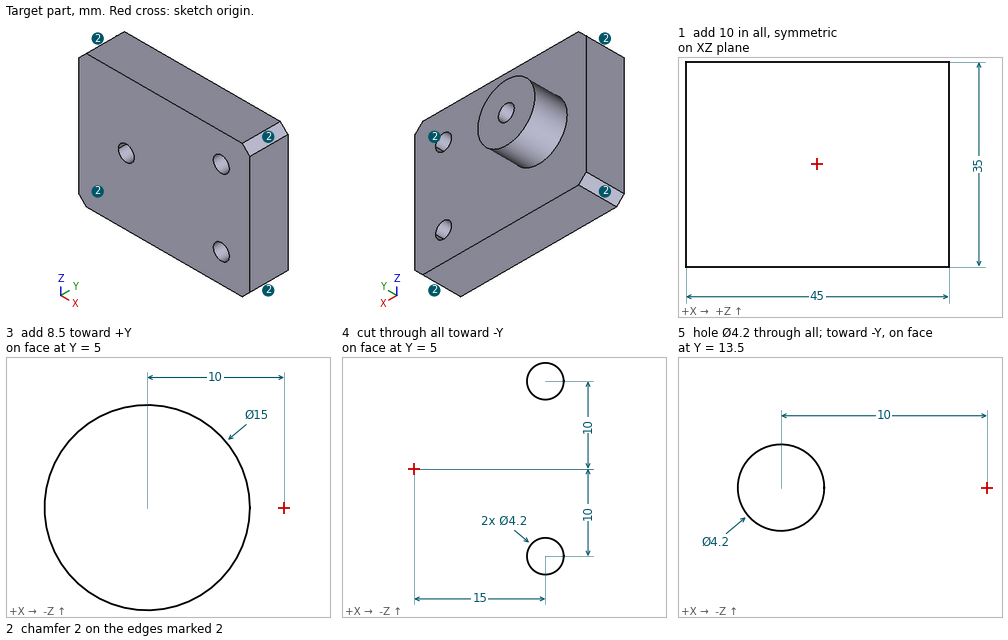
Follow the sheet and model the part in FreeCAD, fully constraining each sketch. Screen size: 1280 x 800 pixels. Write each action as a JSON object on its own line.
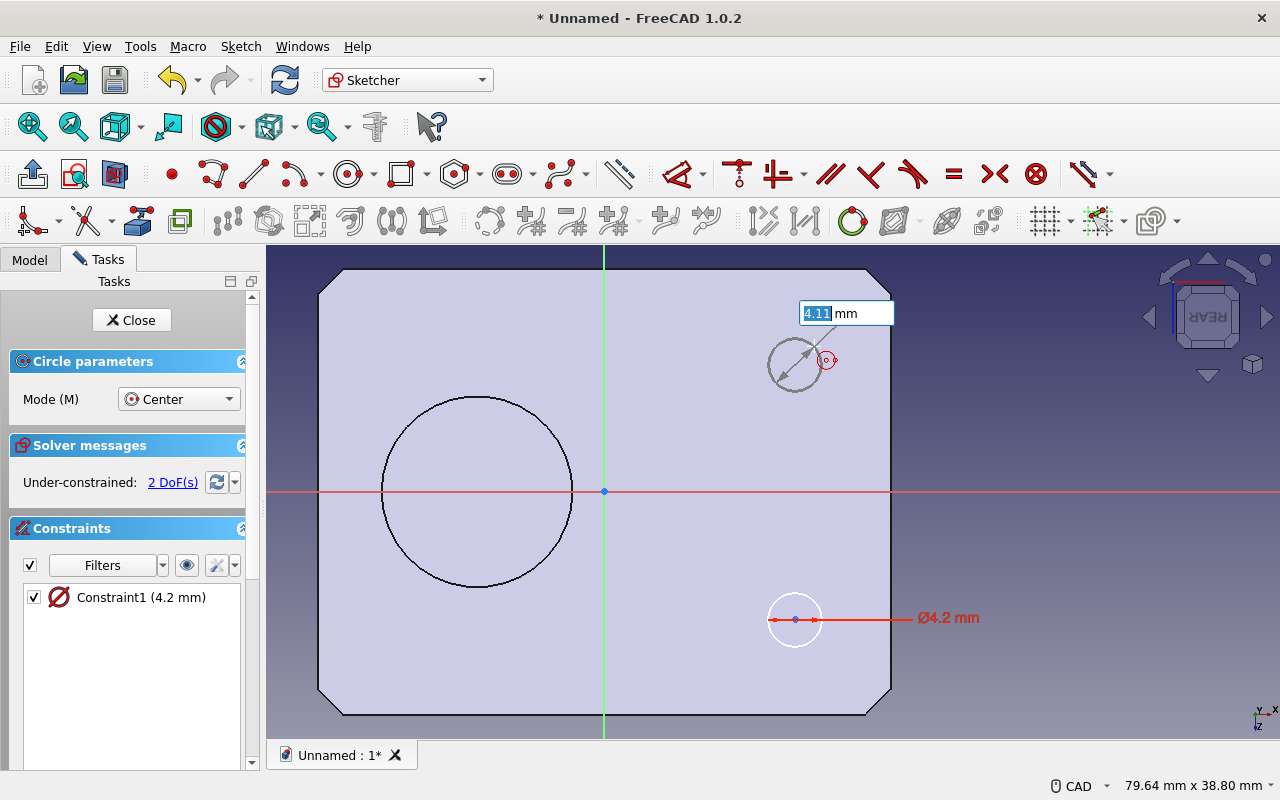
{"action": "type", "text": "4.2"}
{"action": "key", "text": "Return"}
{"action": "key", "text": "Escape"}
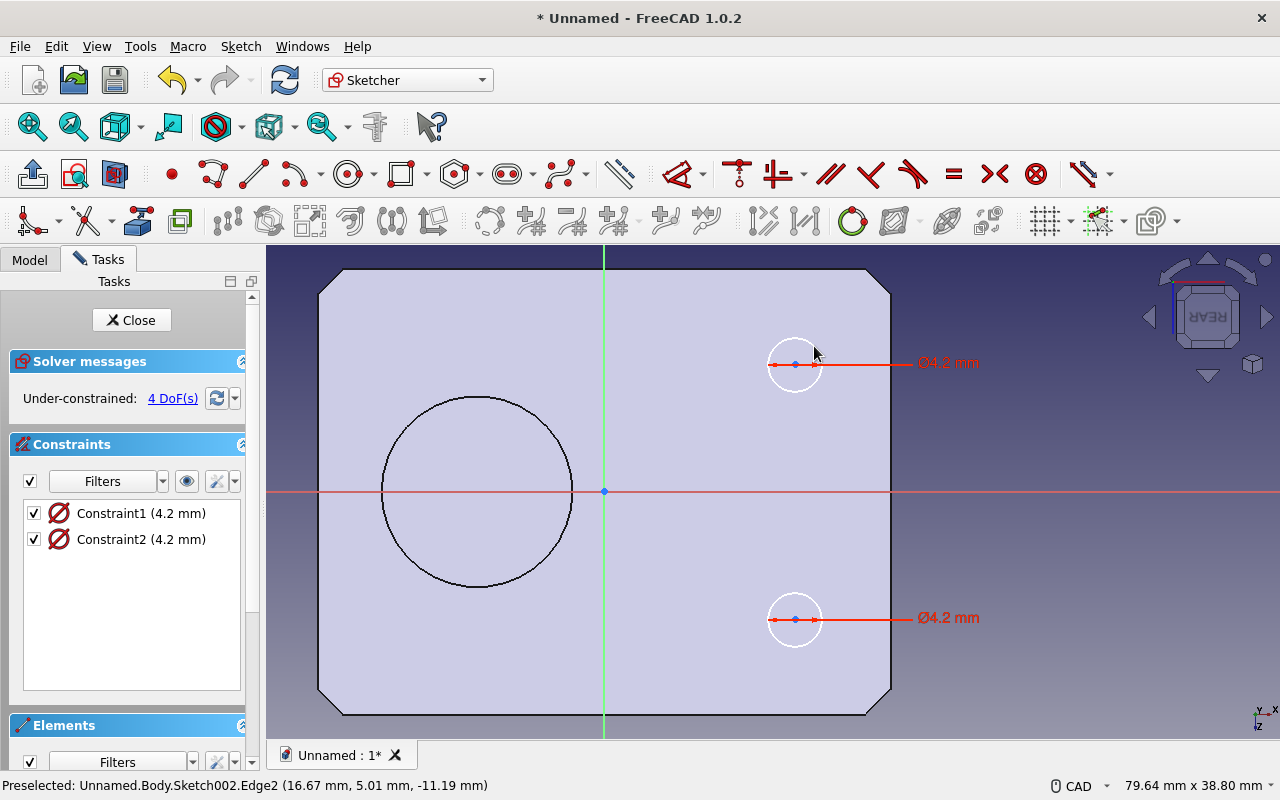
{"action": "left_click", "coordinate": [795, 620]}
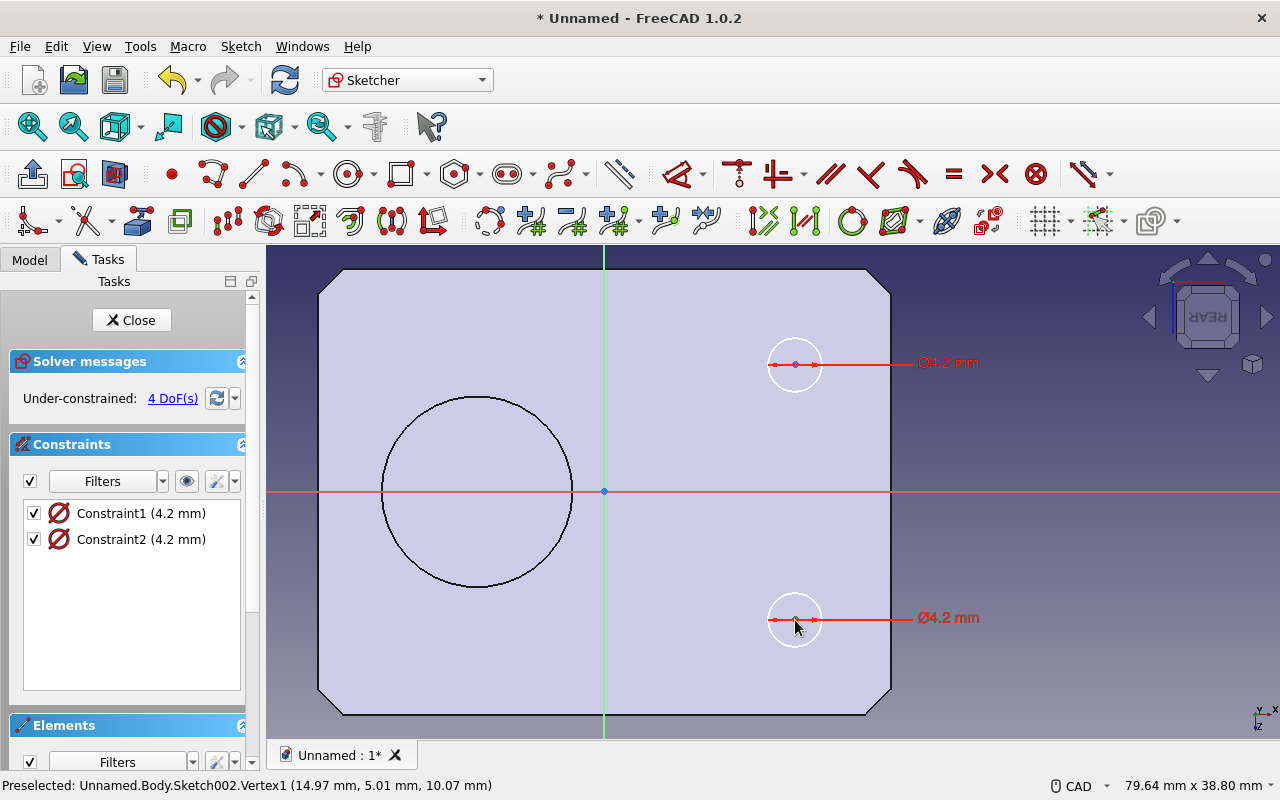
{"action": "left_click", "coordinate": [795, 365]}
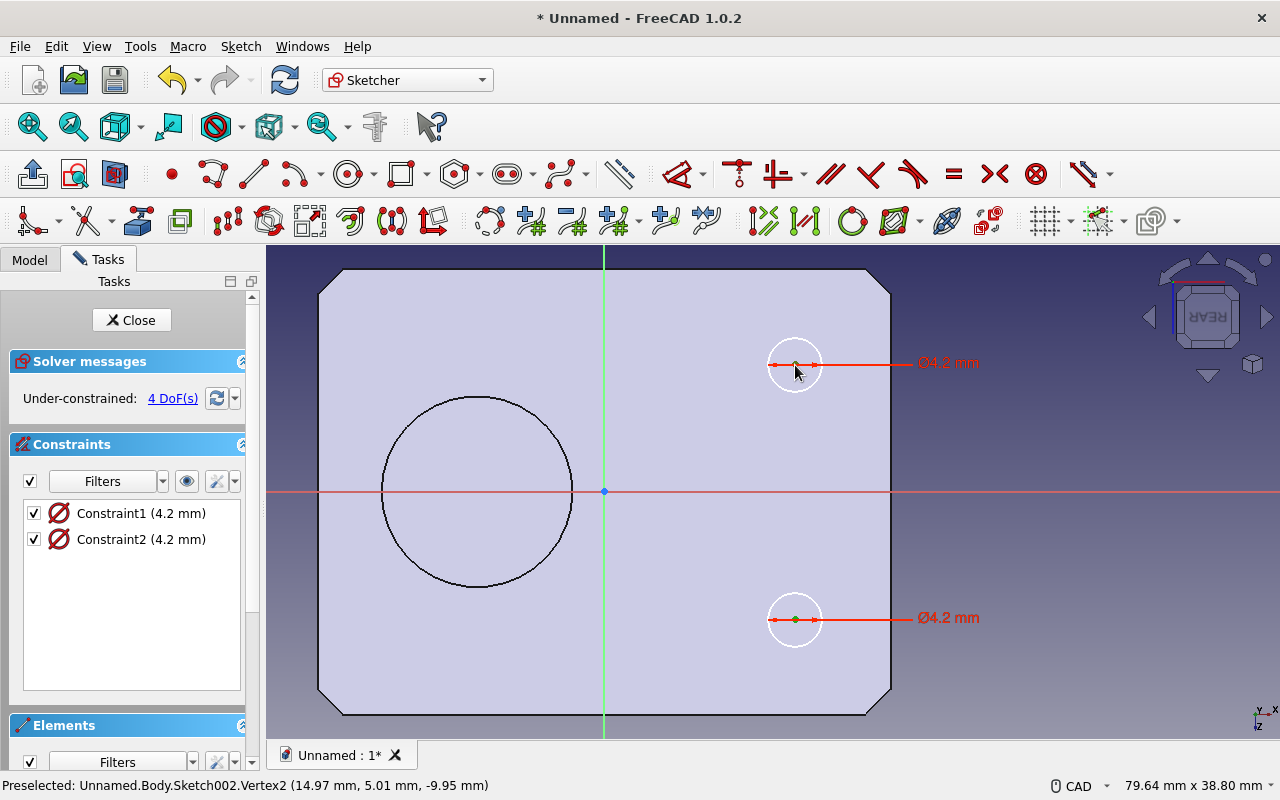
{"action": "left_click", "coordinate": [804, 174]}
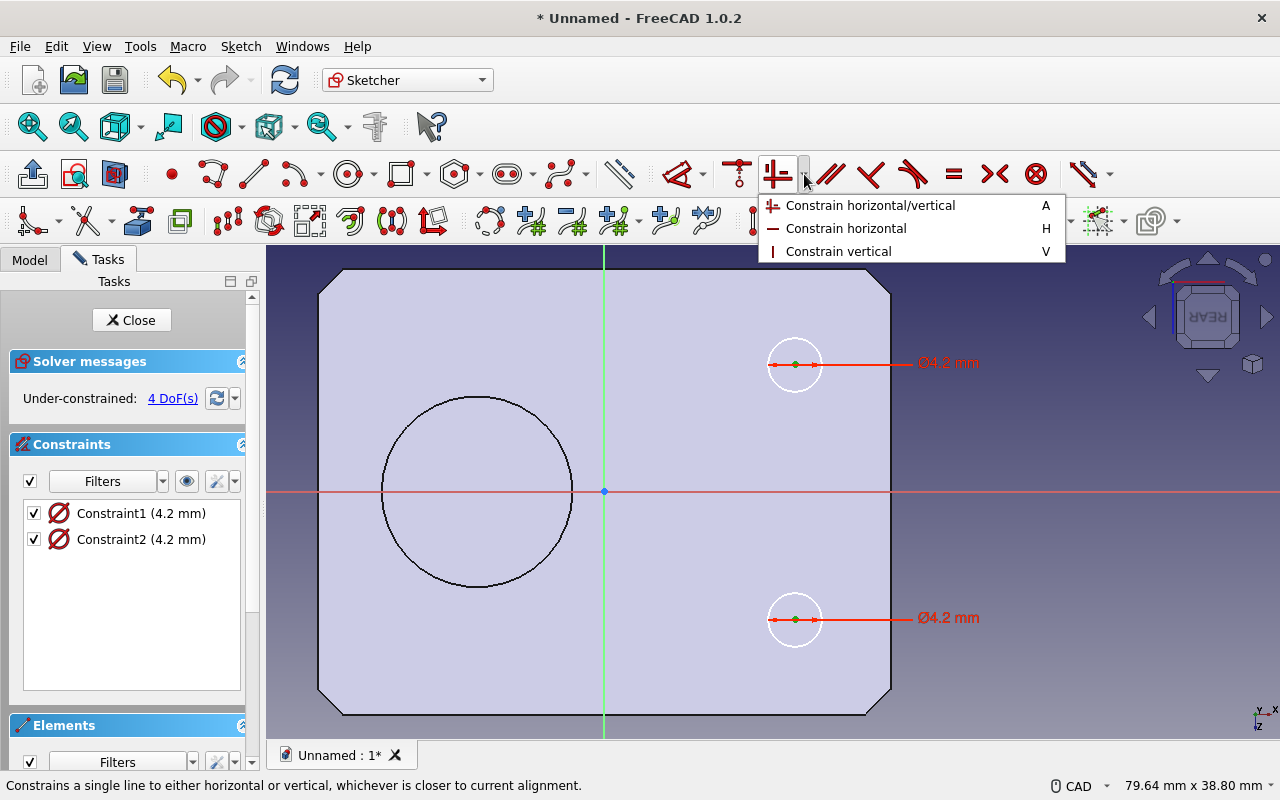
{"action": "left_click", "coordinate": [912, 252]}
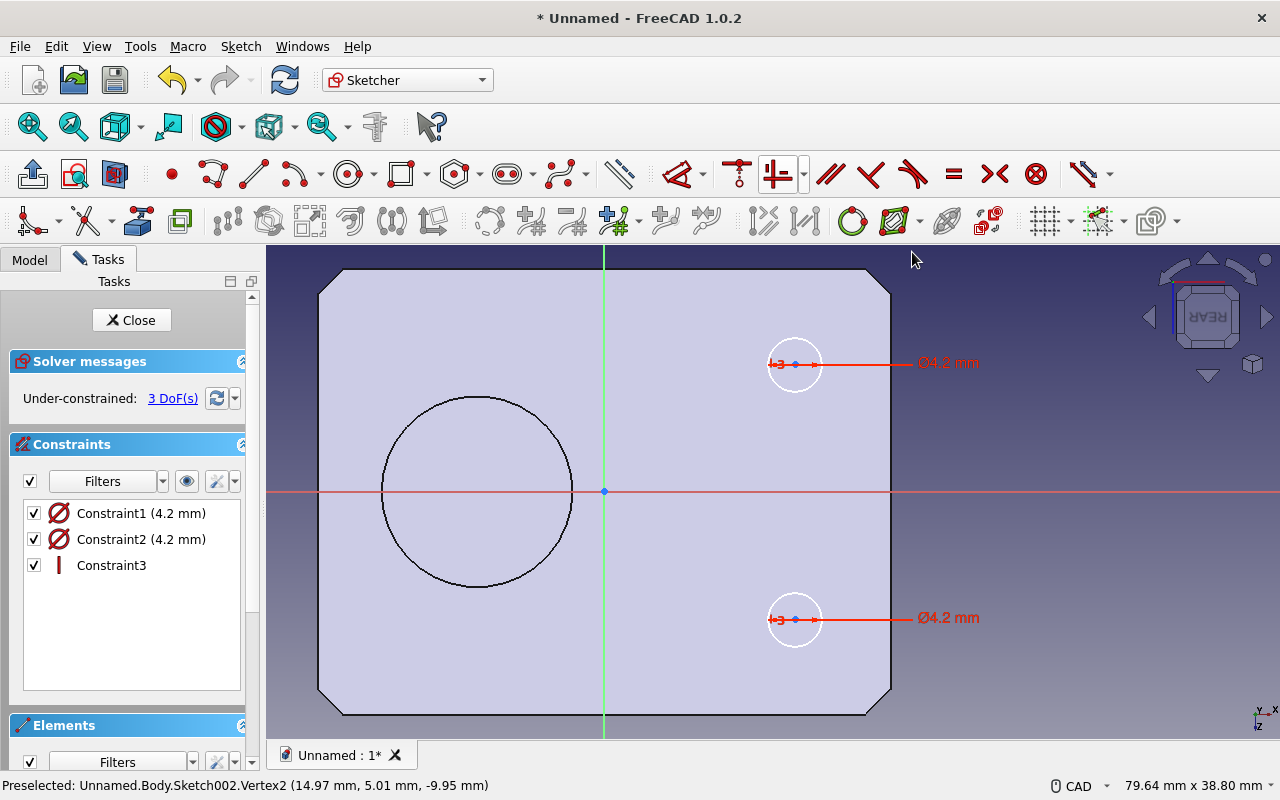
{"action": "key", "text": "d"}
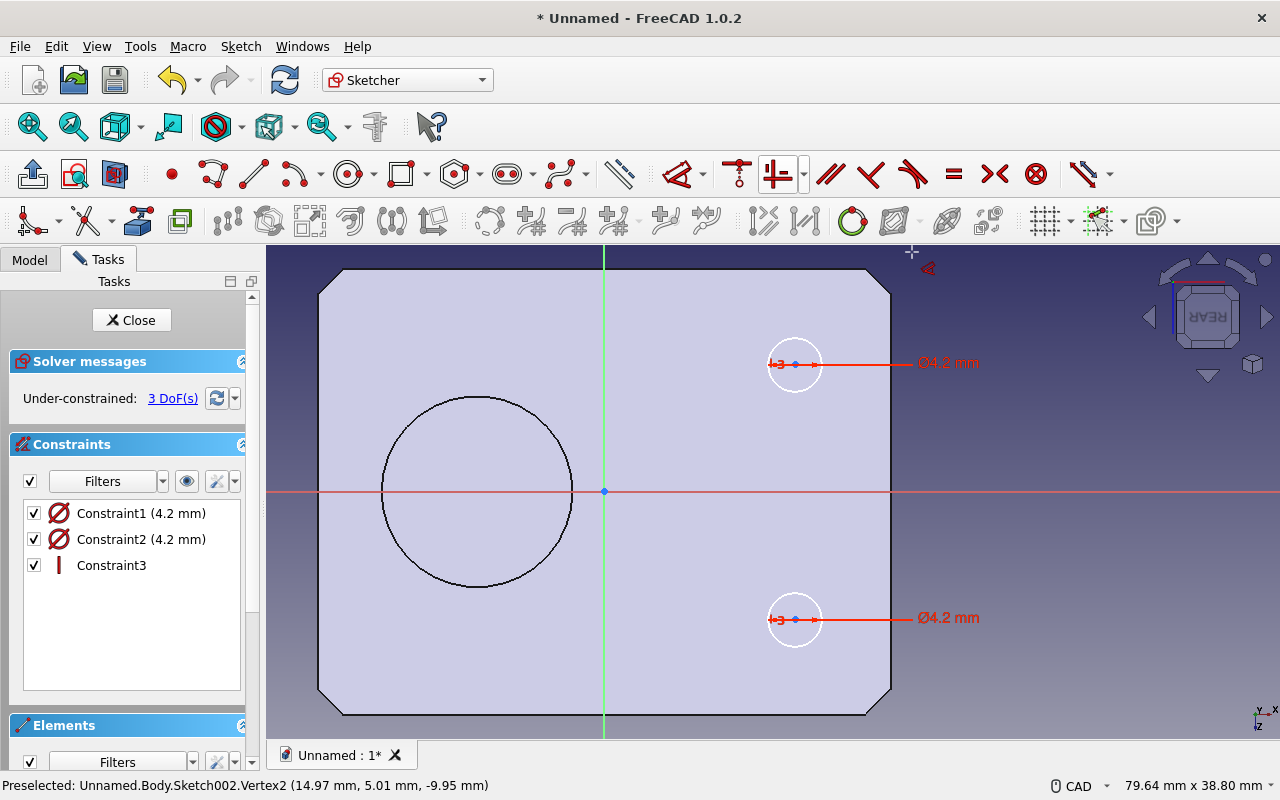
{"action": "left_click", "coordinate": [795, 620]}
{"action": "left_click", "coordinate": [700, 654]}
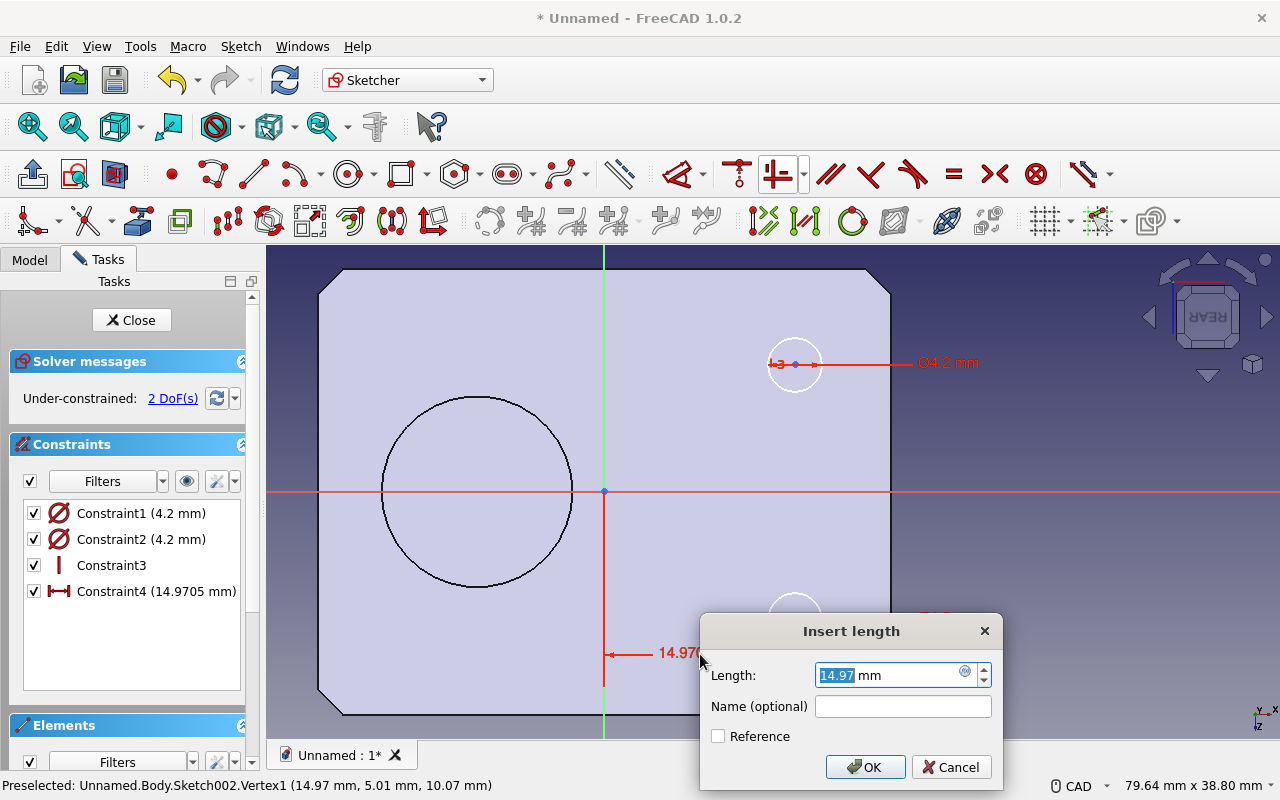
{"action": "type", "text": "15"}
{"action": "key", "text": "Return"}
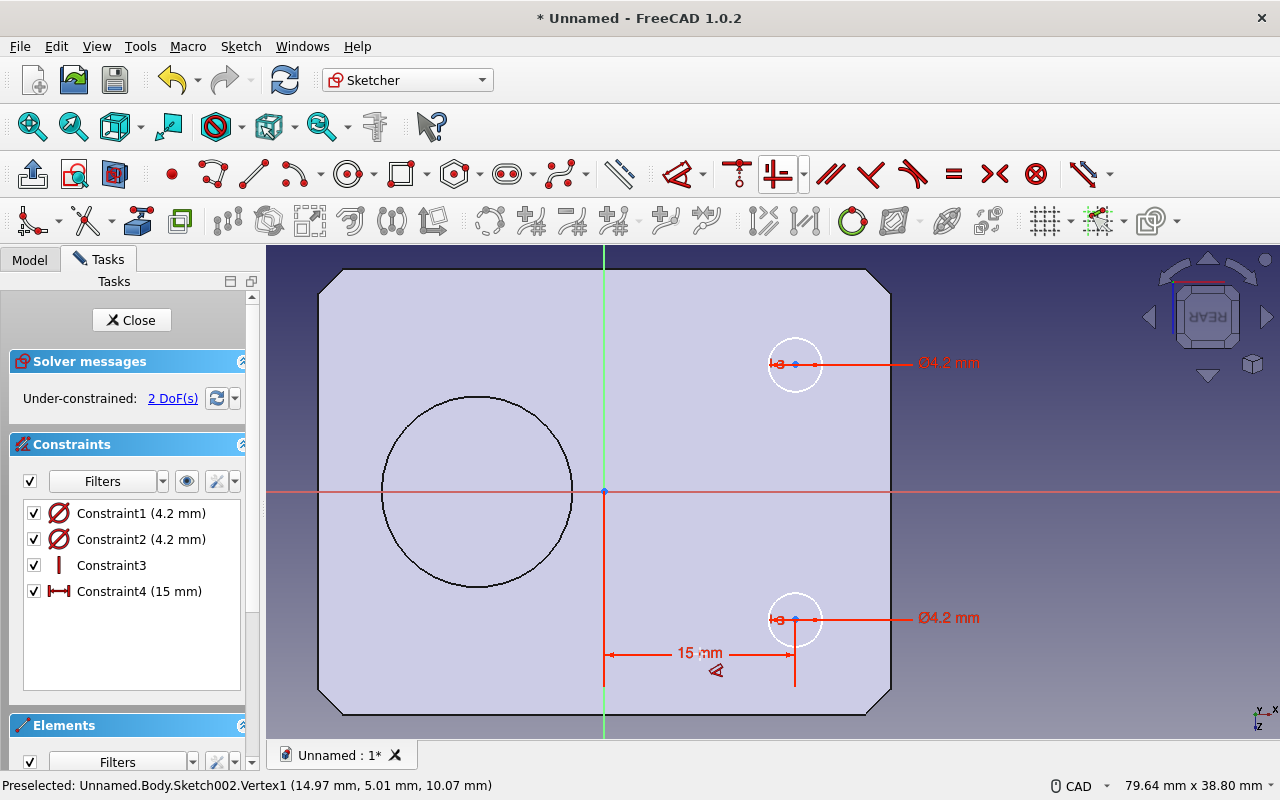
{"action": "left_click", "coordinate": [795, 620]}
{"action": "left_click", "coordinate": [570, 556]}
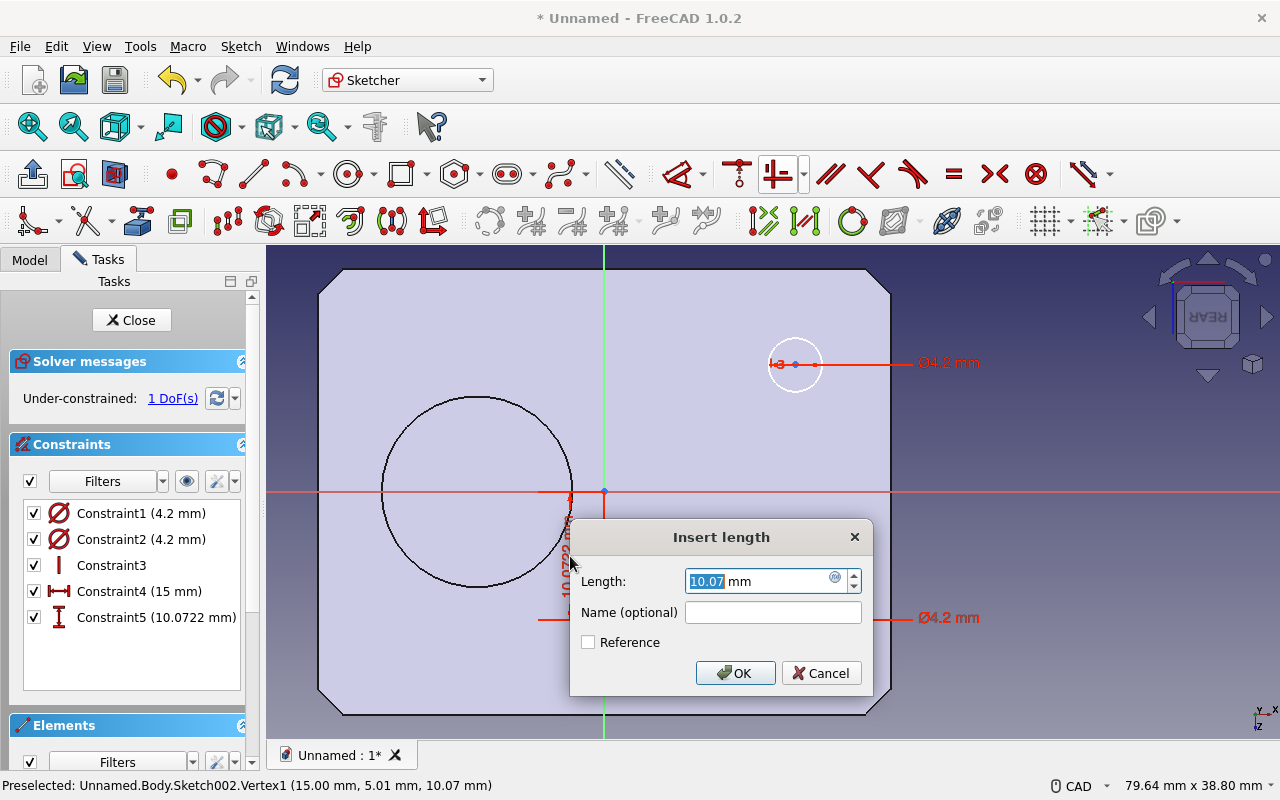
{"action": "type", "text": "10"}
{"action": "key", "text": "Return"}